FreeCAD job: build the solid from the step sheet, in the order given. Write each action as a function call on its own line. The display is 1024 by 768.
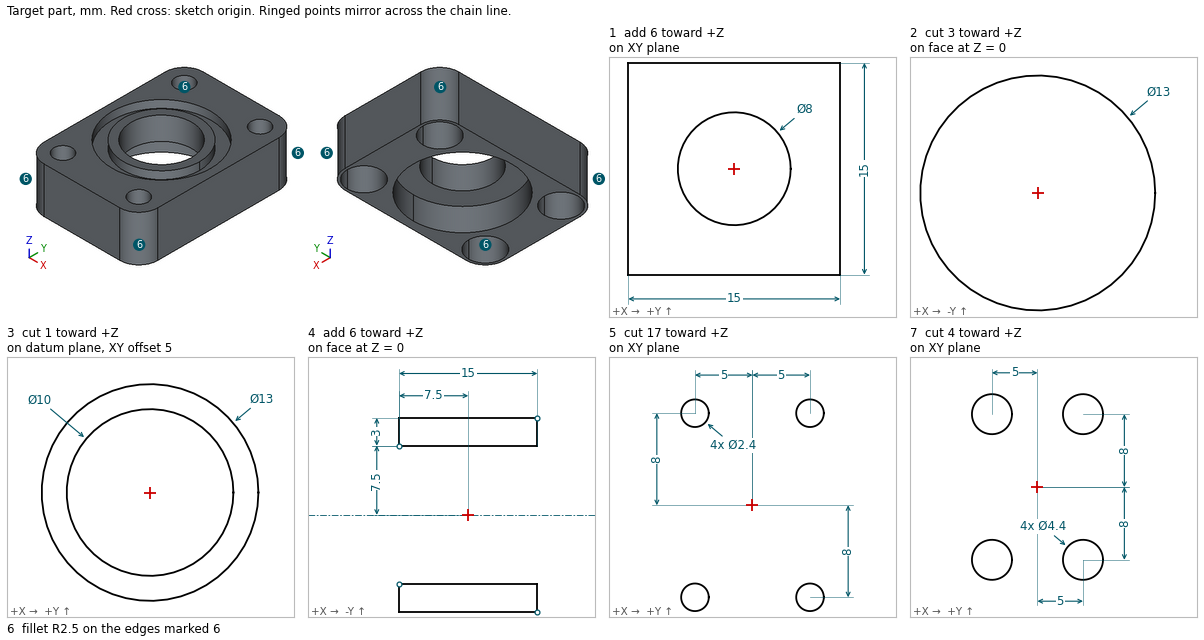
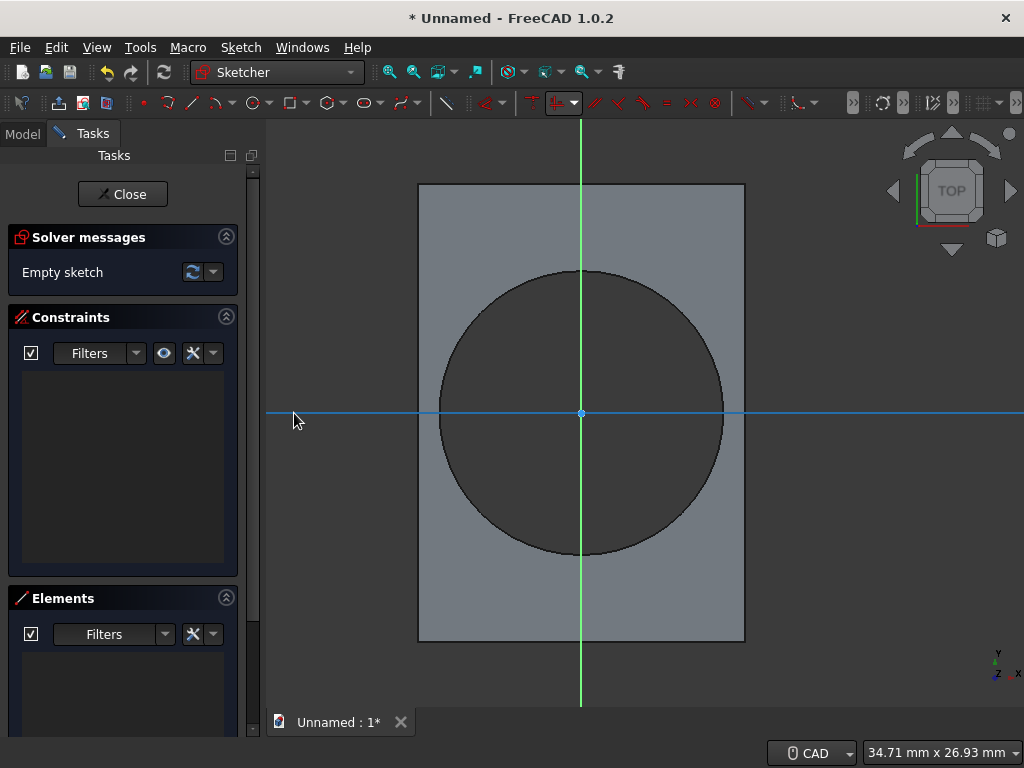
click(254, 104)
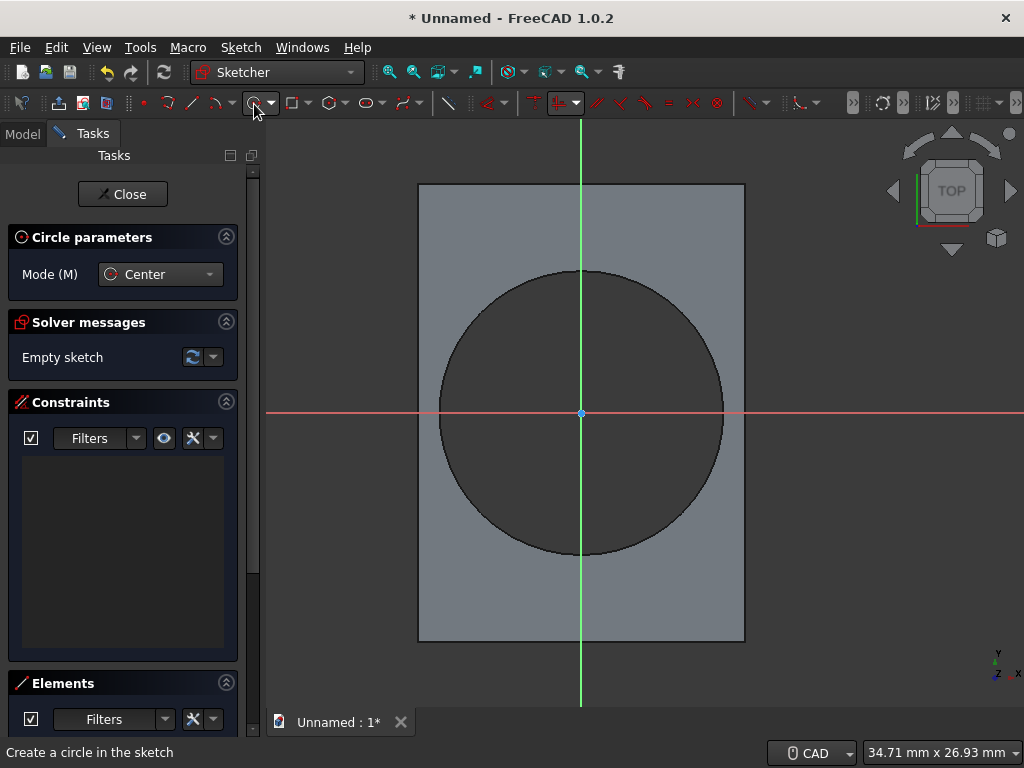
click(472, 238)
click(491, 220)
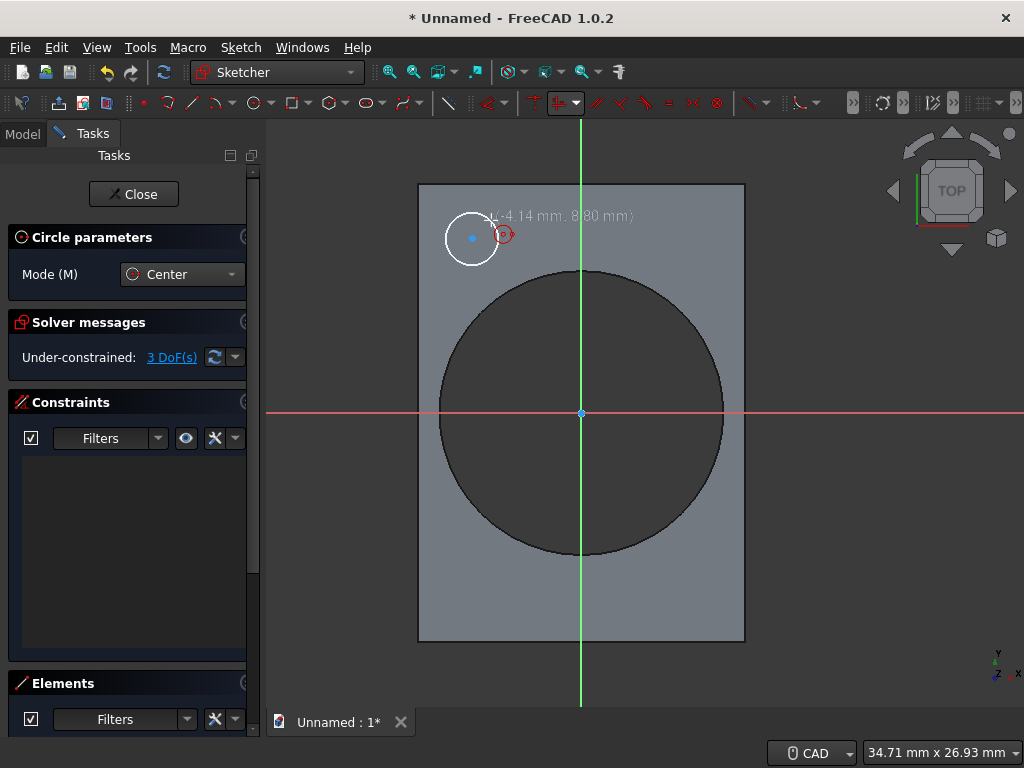
click(691, 238)
click(709, 220)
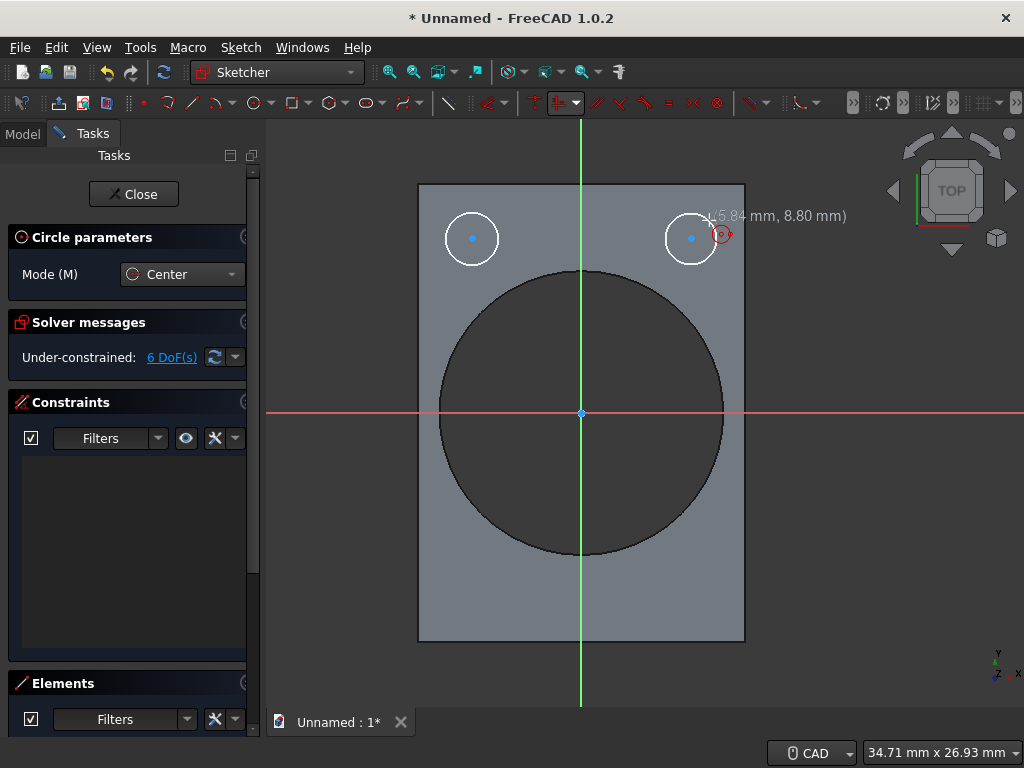
click(691, 588)
click(709, 569)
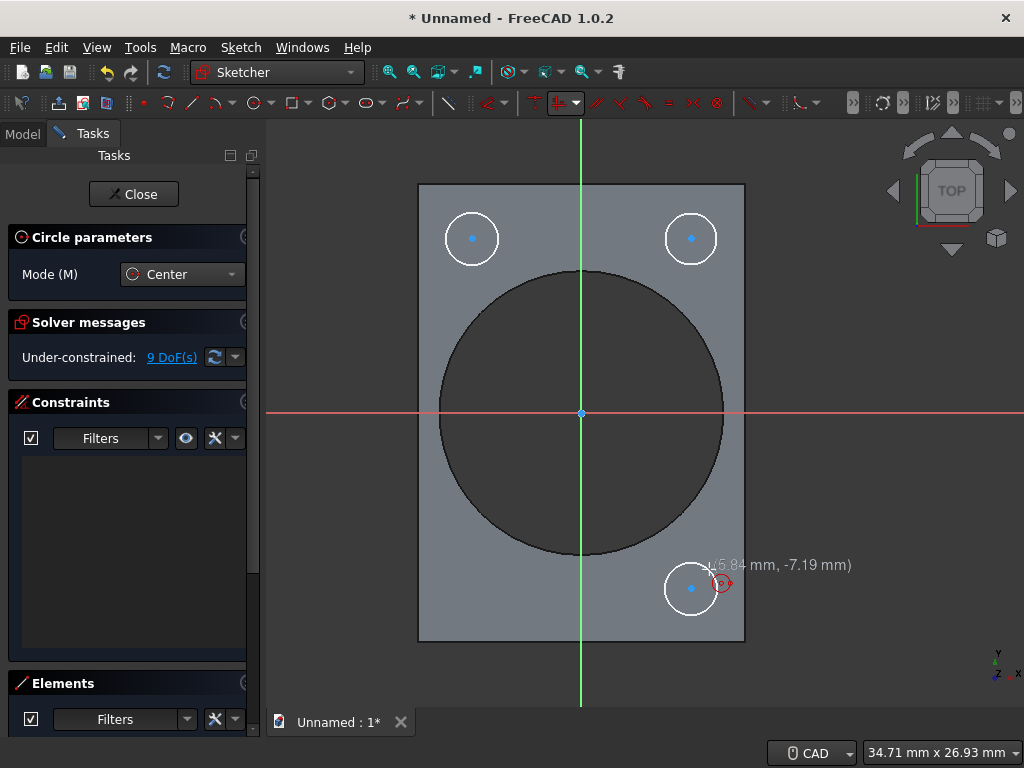
click(472, 588)
click(491, 569)
key(Escape)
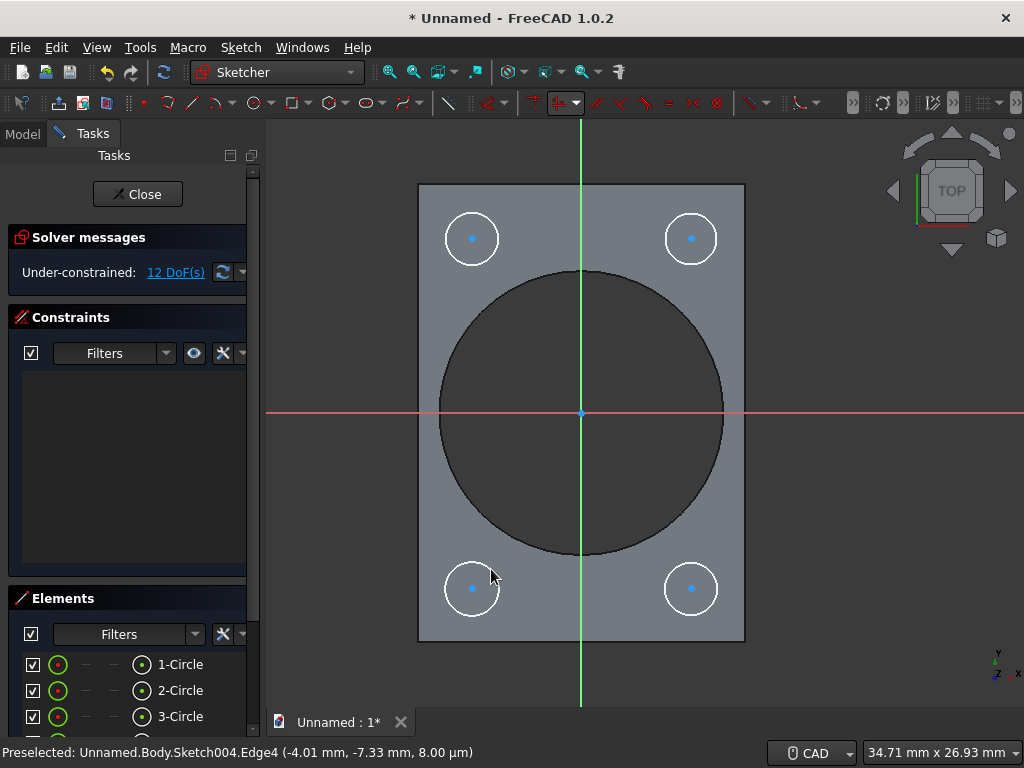
click(490, 220)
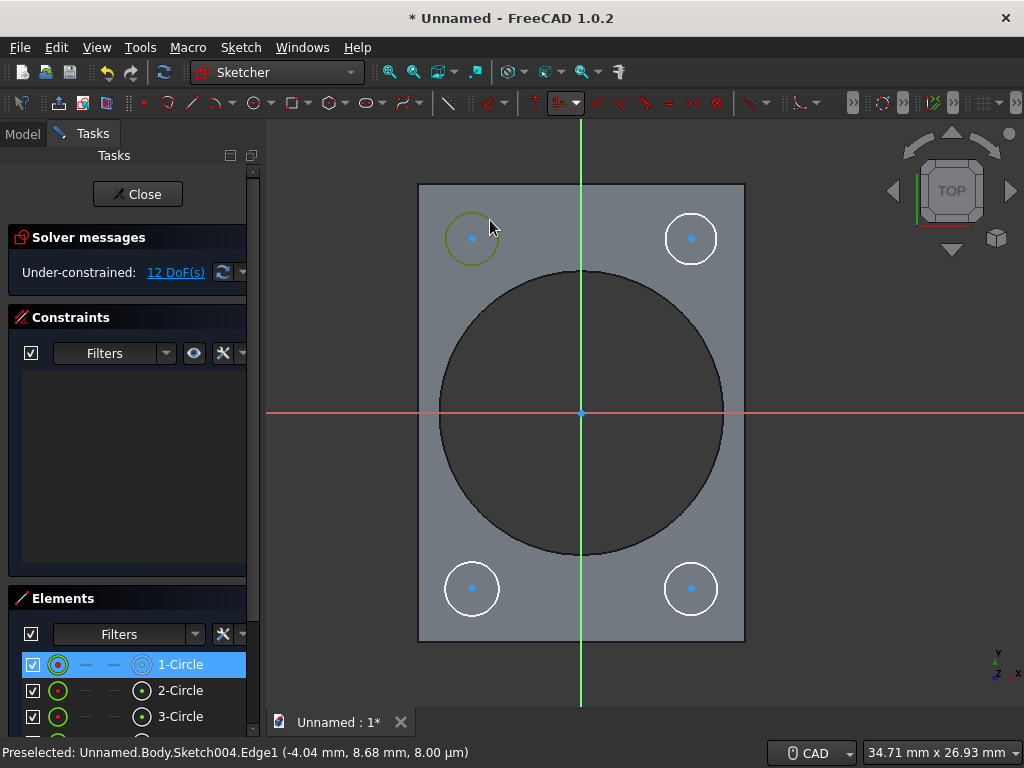
click(709, 221)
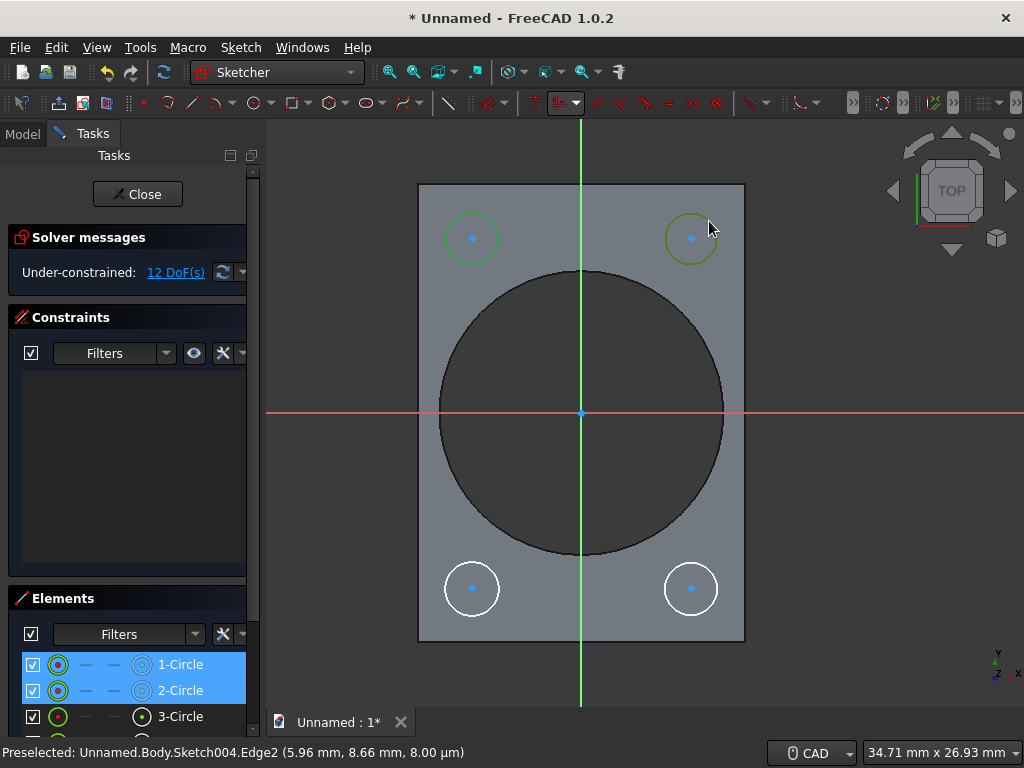
click(709, 570)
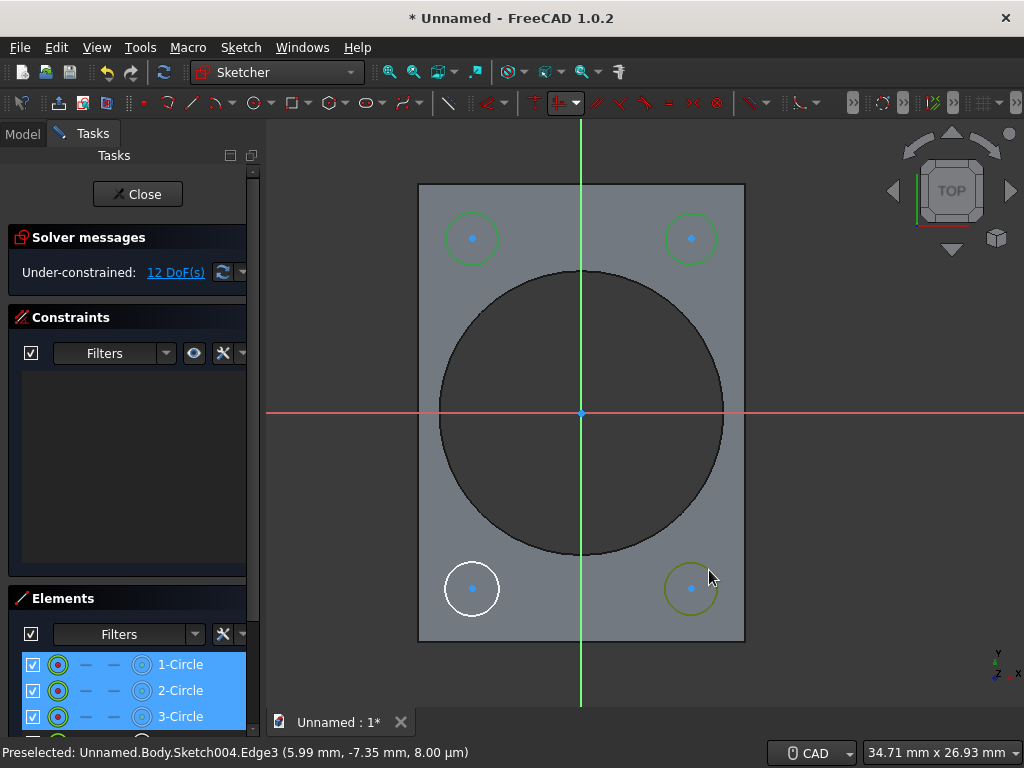
click(491, 570)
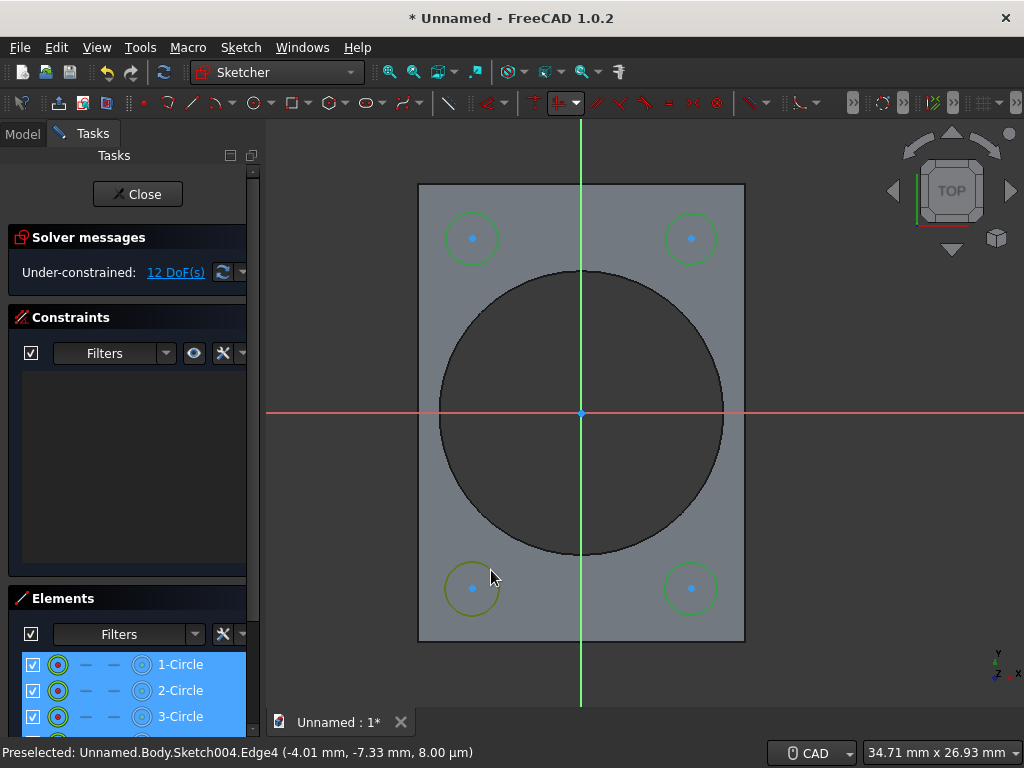
key(e)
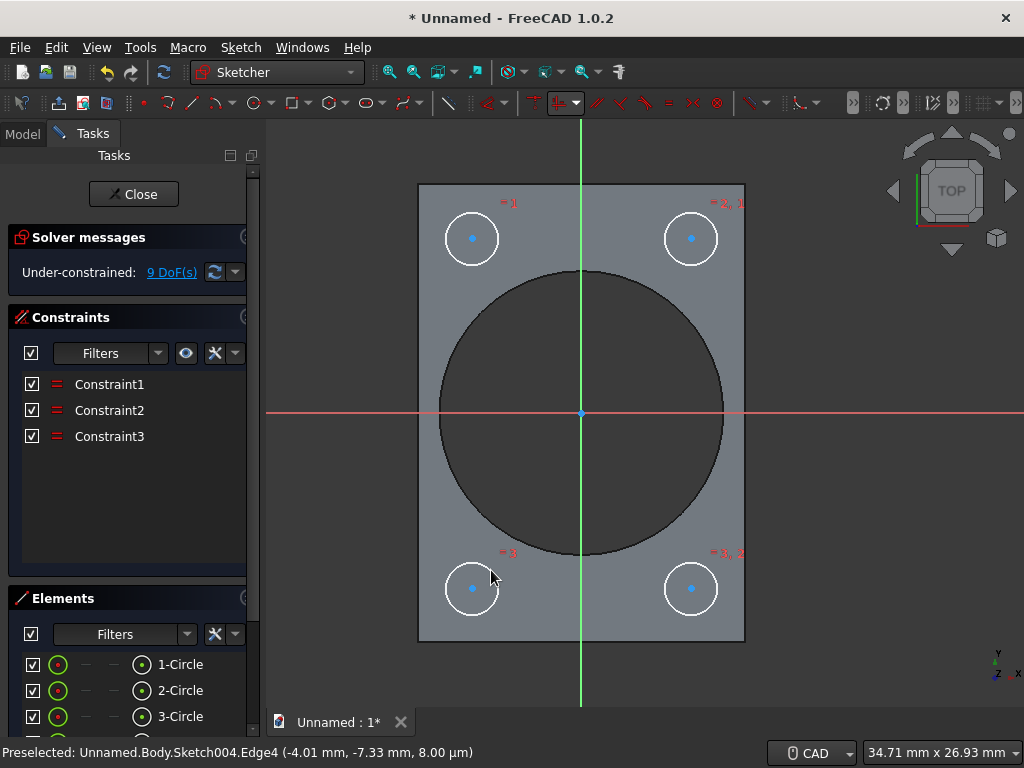
click(472, 239)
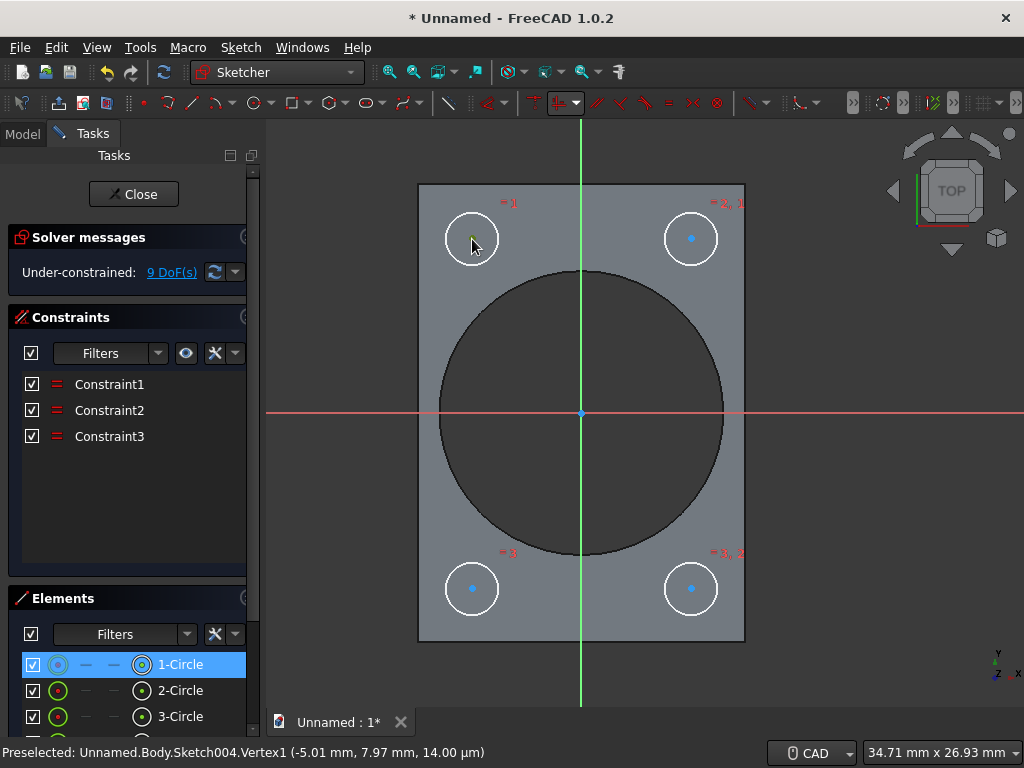
click(691, 239)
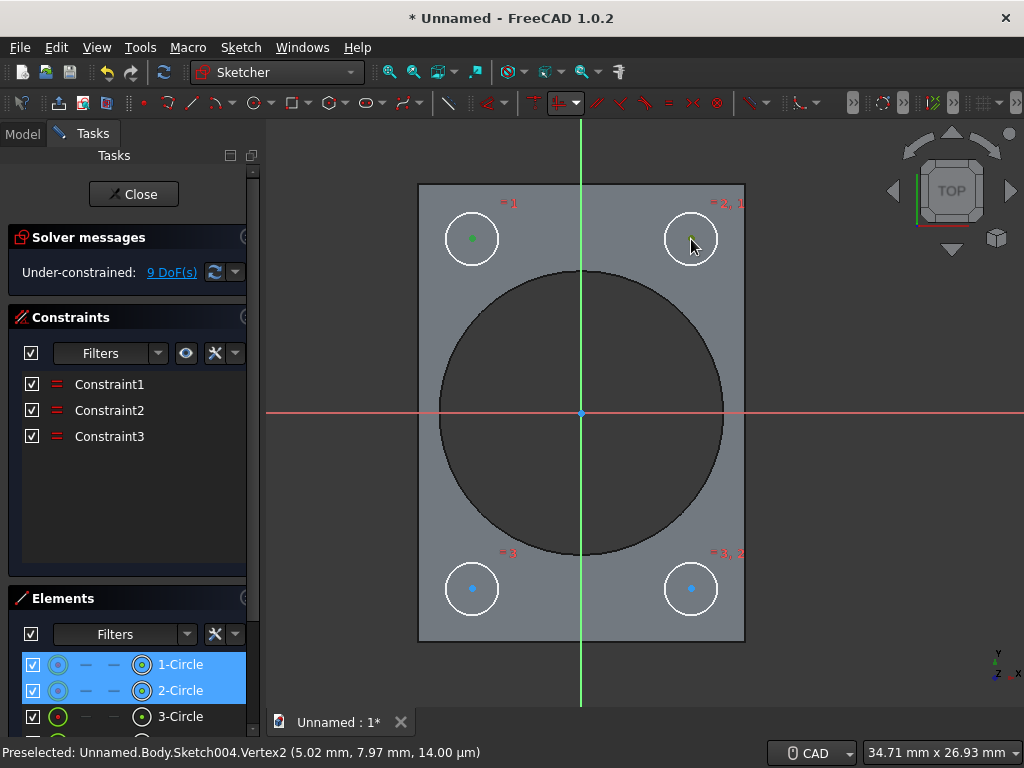
click(578, 104)